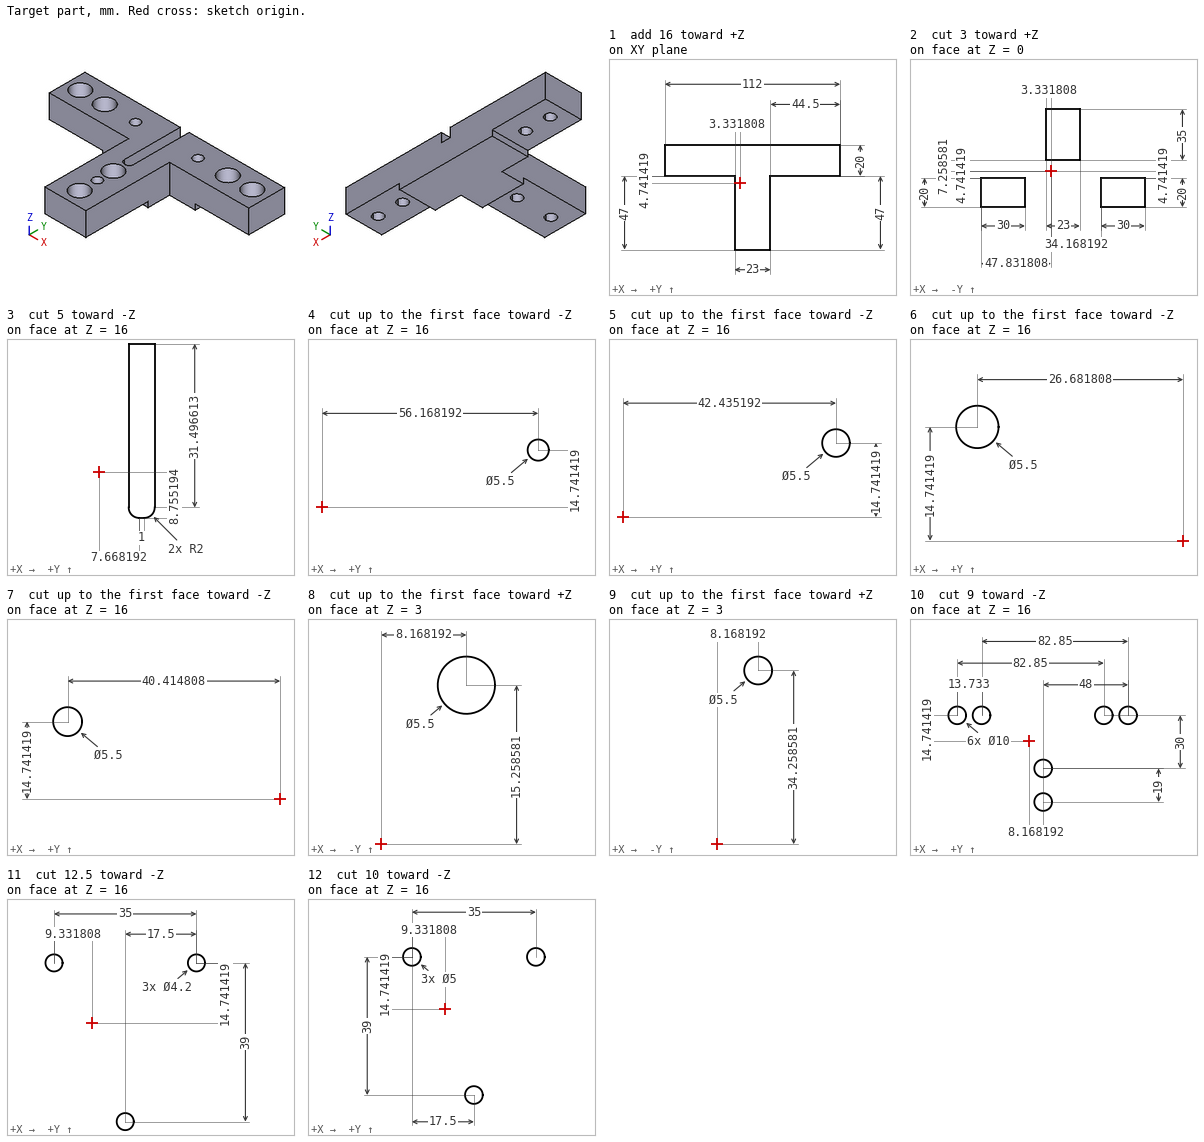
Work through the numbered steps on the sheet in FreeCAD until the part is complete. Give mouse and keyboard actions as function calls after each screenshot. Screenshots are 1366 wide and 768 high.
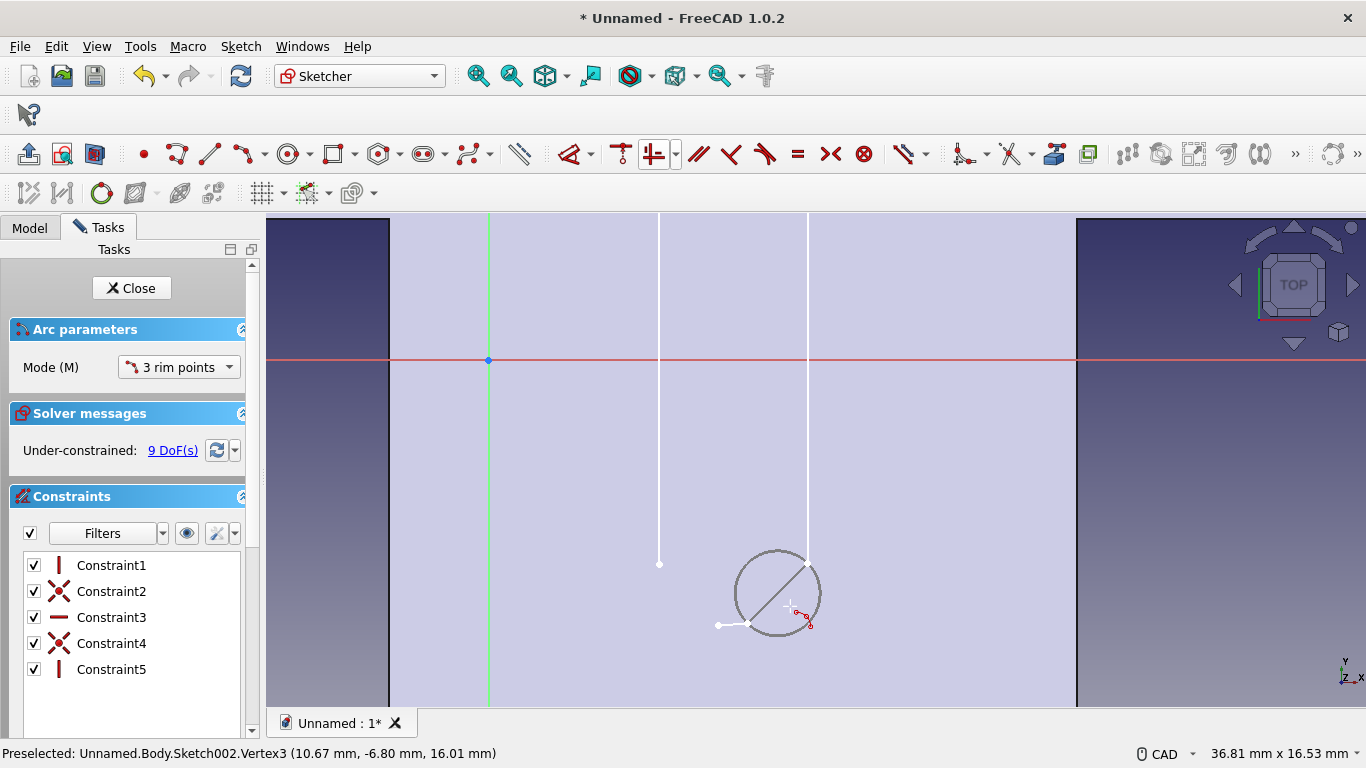
click(790, 604)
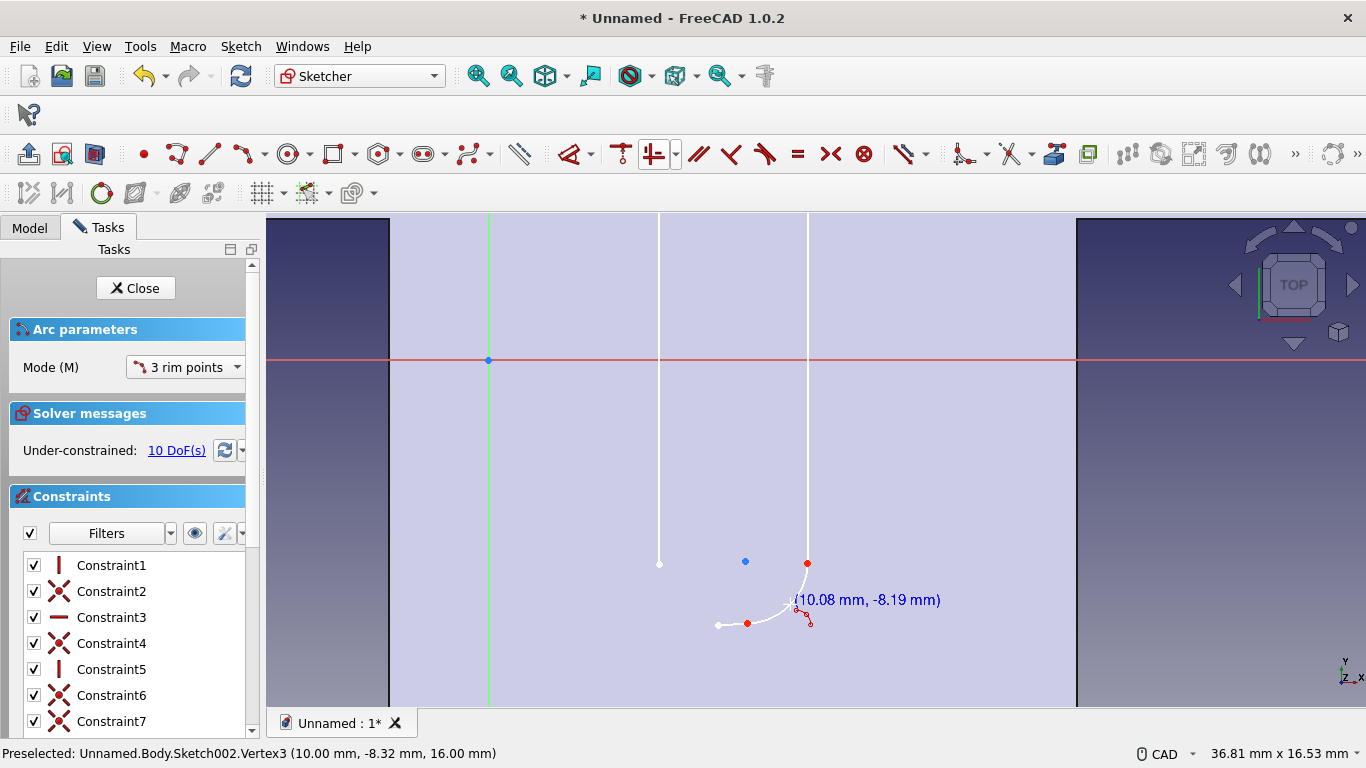
click(659, 564)
click(719, 626)
click(676, 604)
key(Escape)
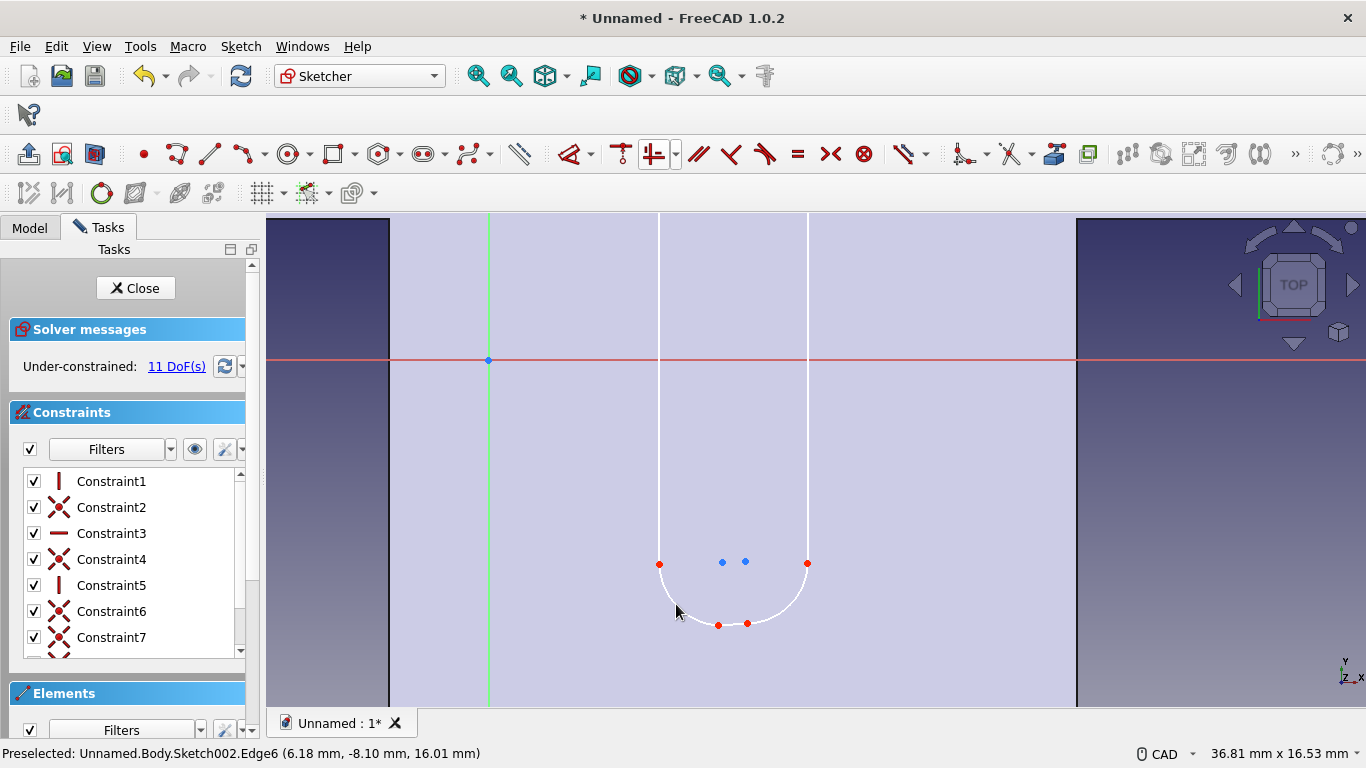
click(730, 625)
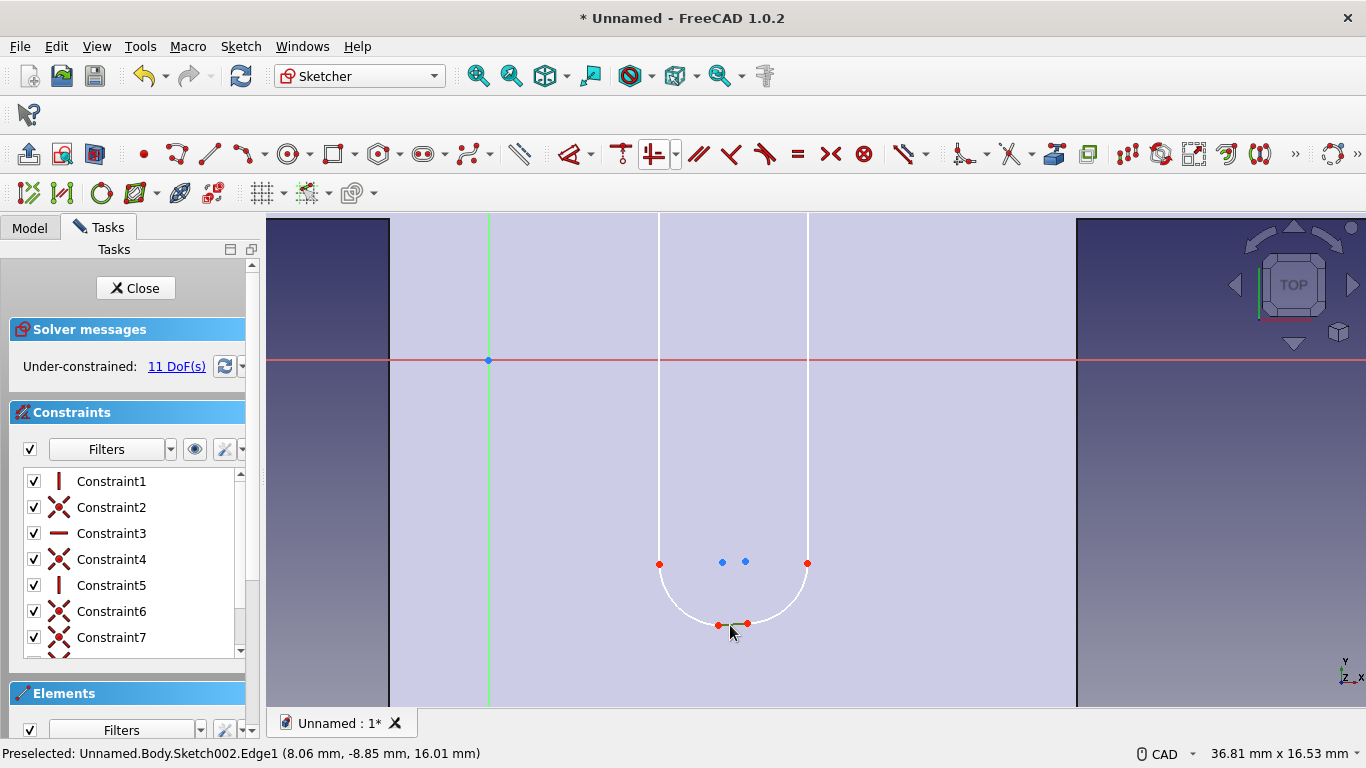
click(775, 616)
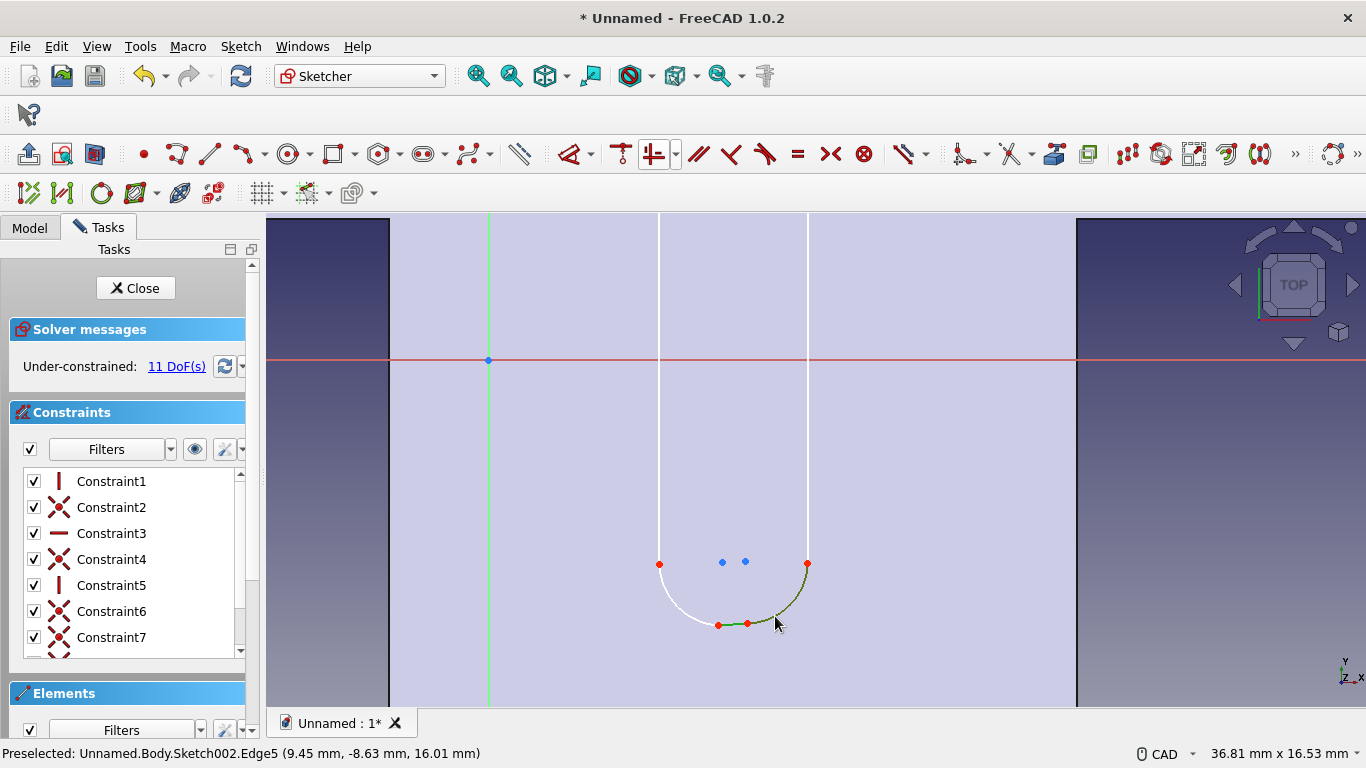
click(765, 154)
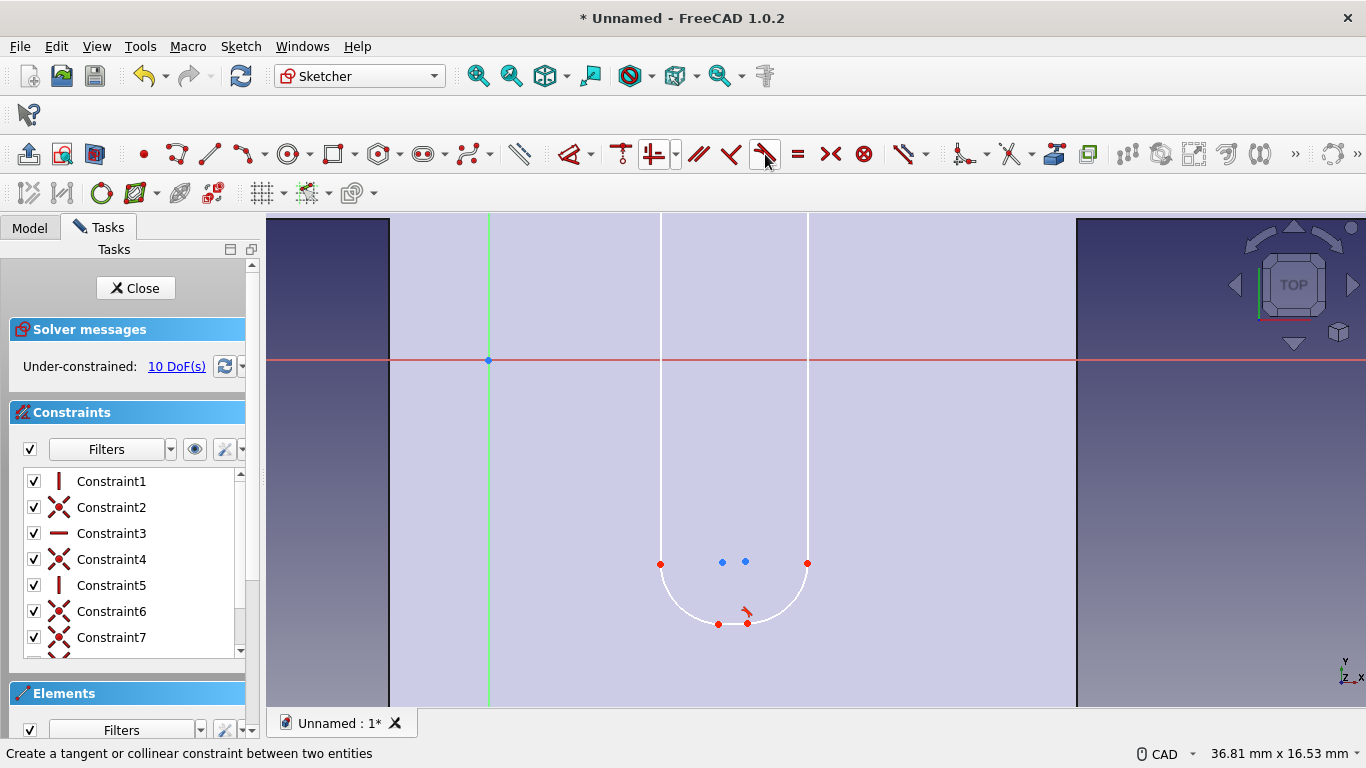
click(730, 624)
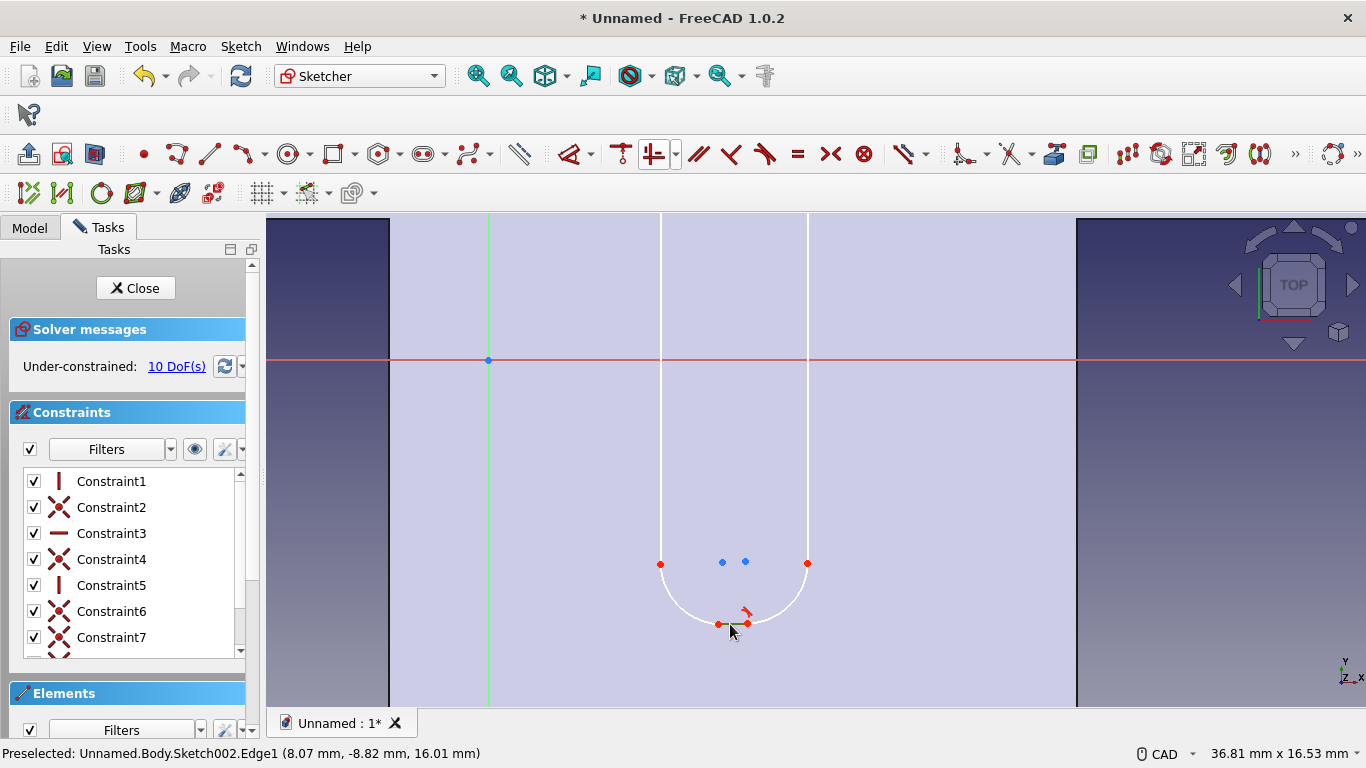
click(668, 591)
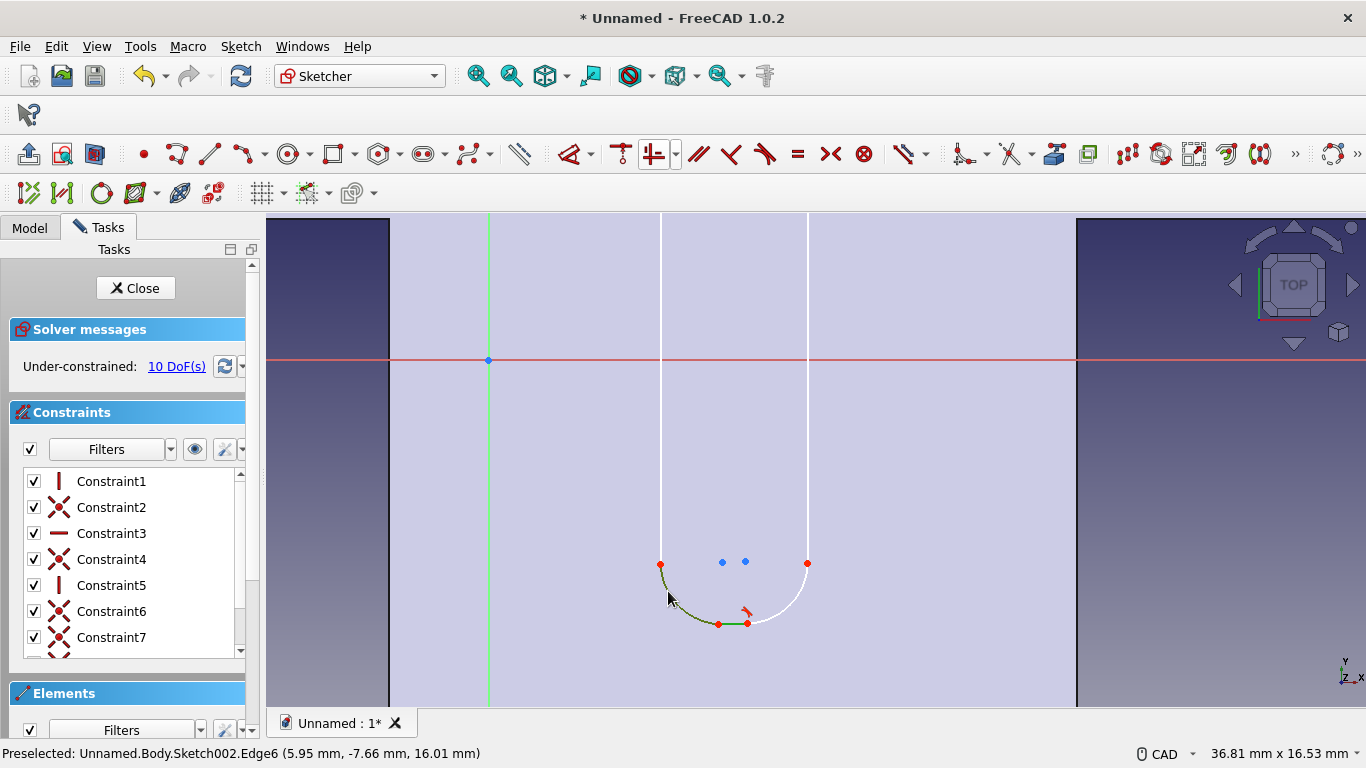
click(765, 154)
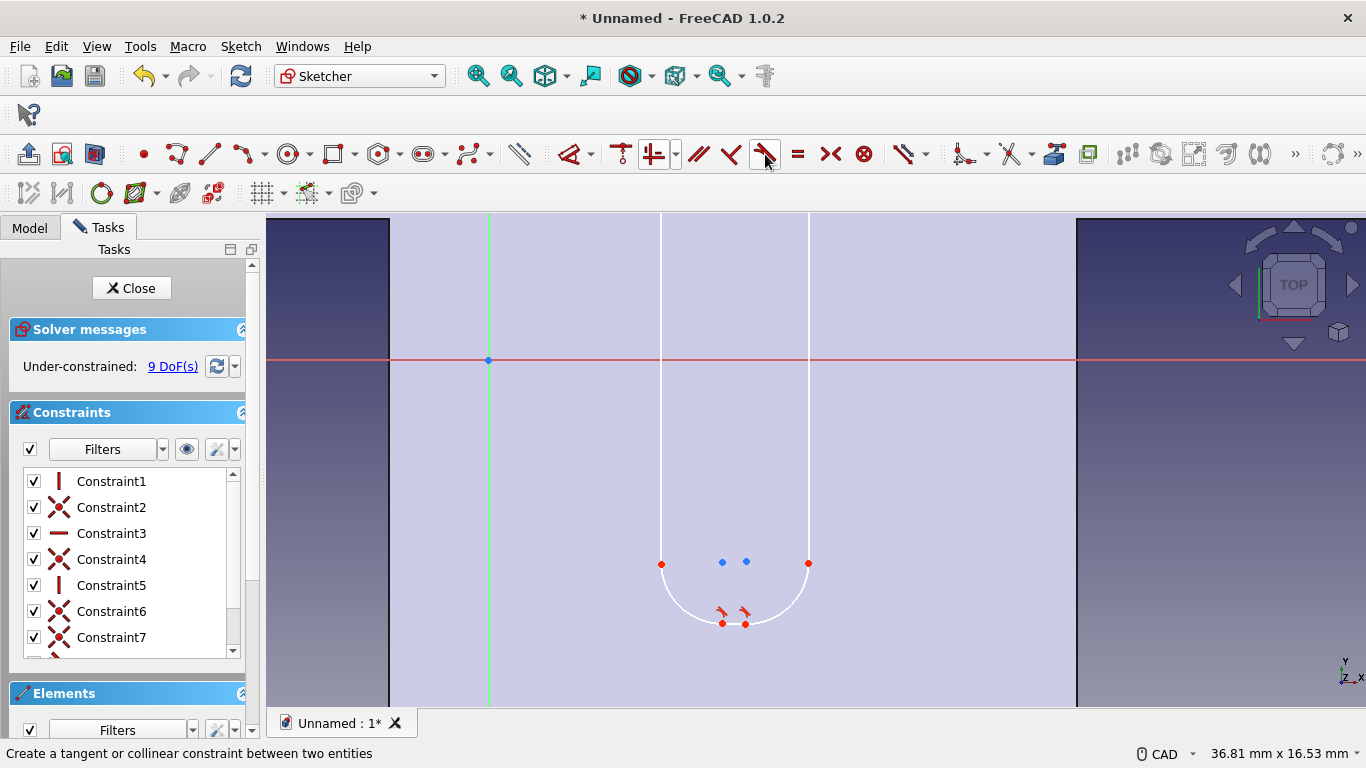
click(809, 282)